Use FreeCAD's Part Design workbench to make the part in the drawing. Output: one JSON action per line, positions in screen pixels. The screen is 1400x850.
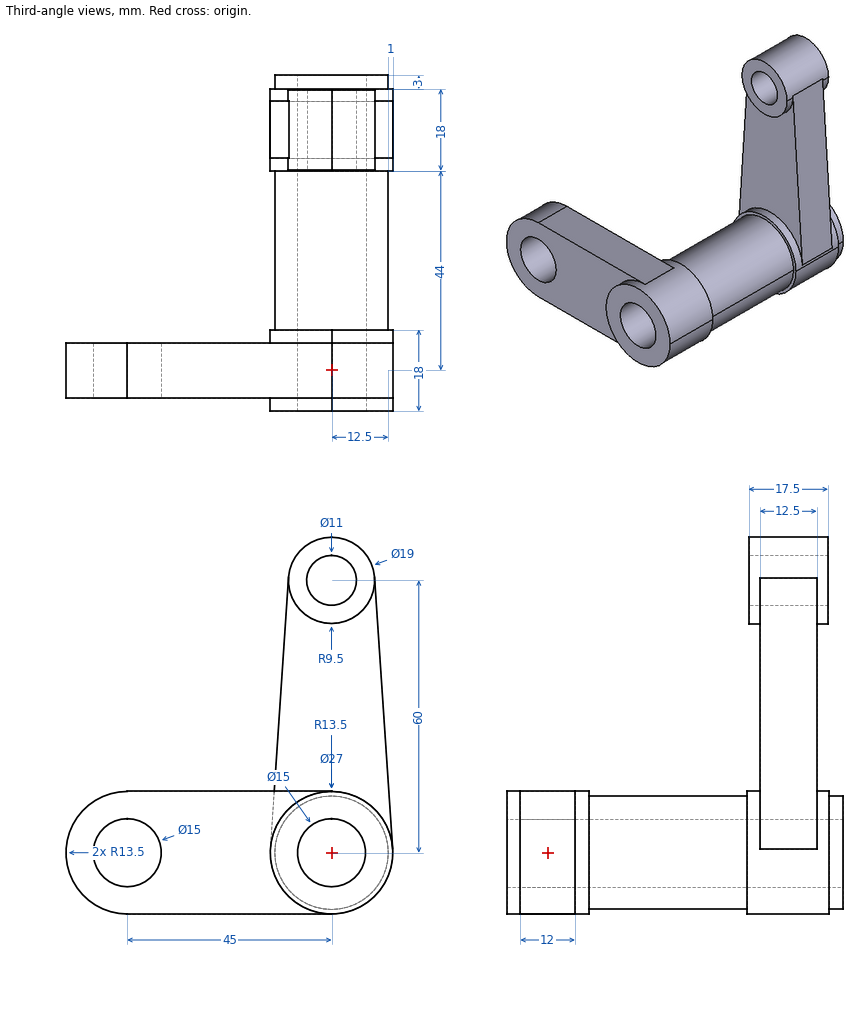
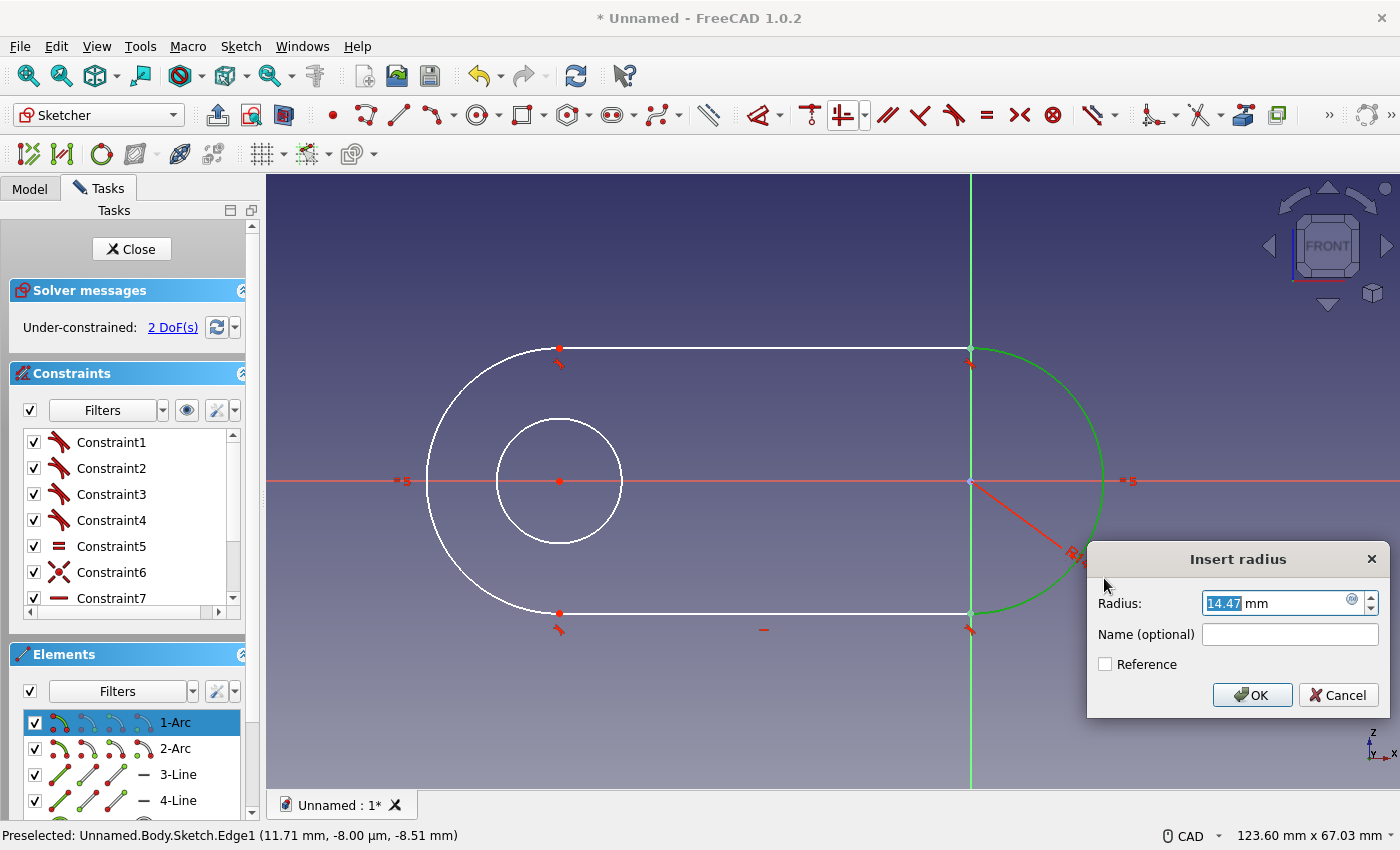
{"action": "type", "text": "13.5"}
{"action": "key", "text": "Return"}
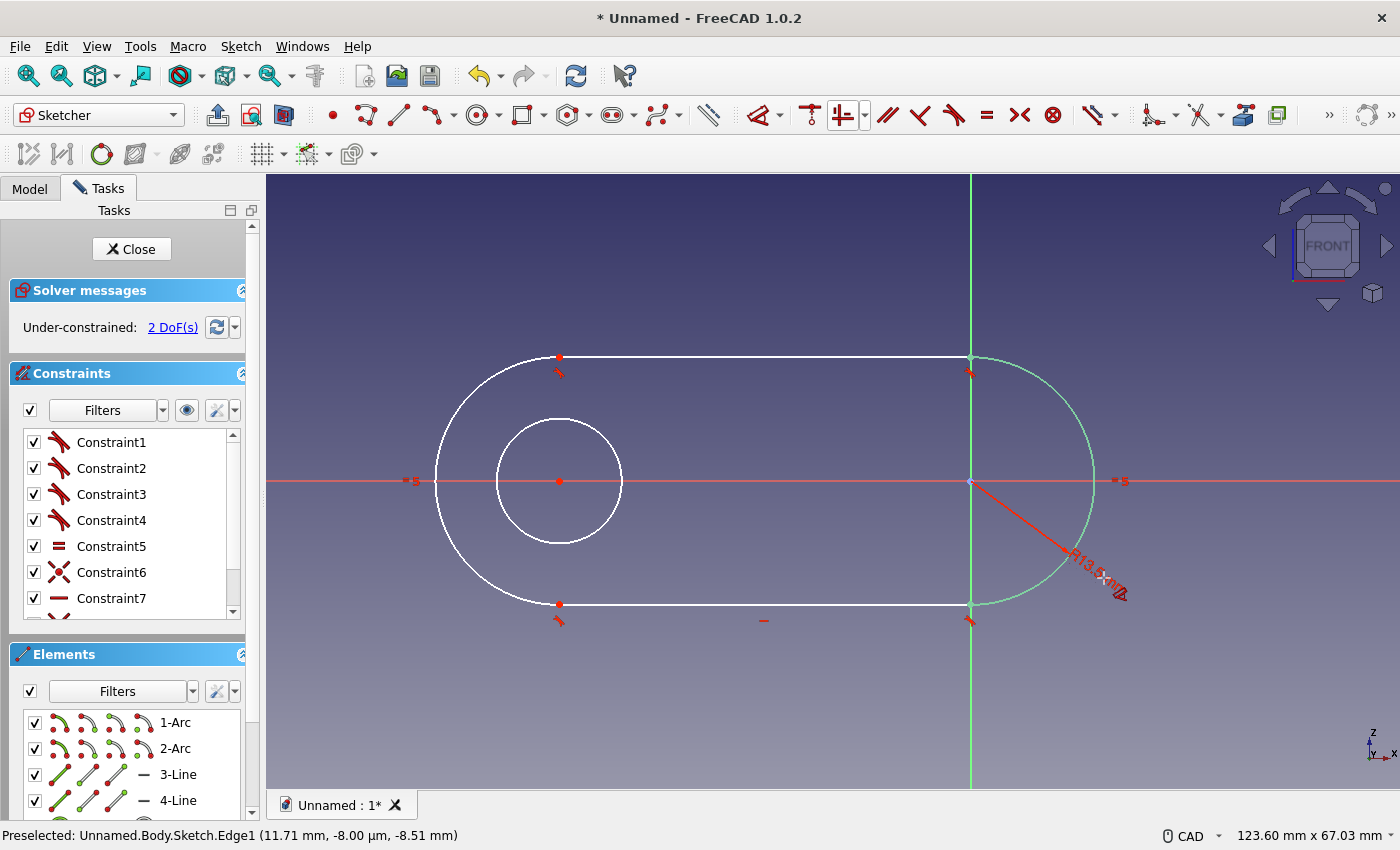
{"action": "left_click", "coordinate": [603, 437]}
{"action": "left_click", "coordinate": [626, 414]}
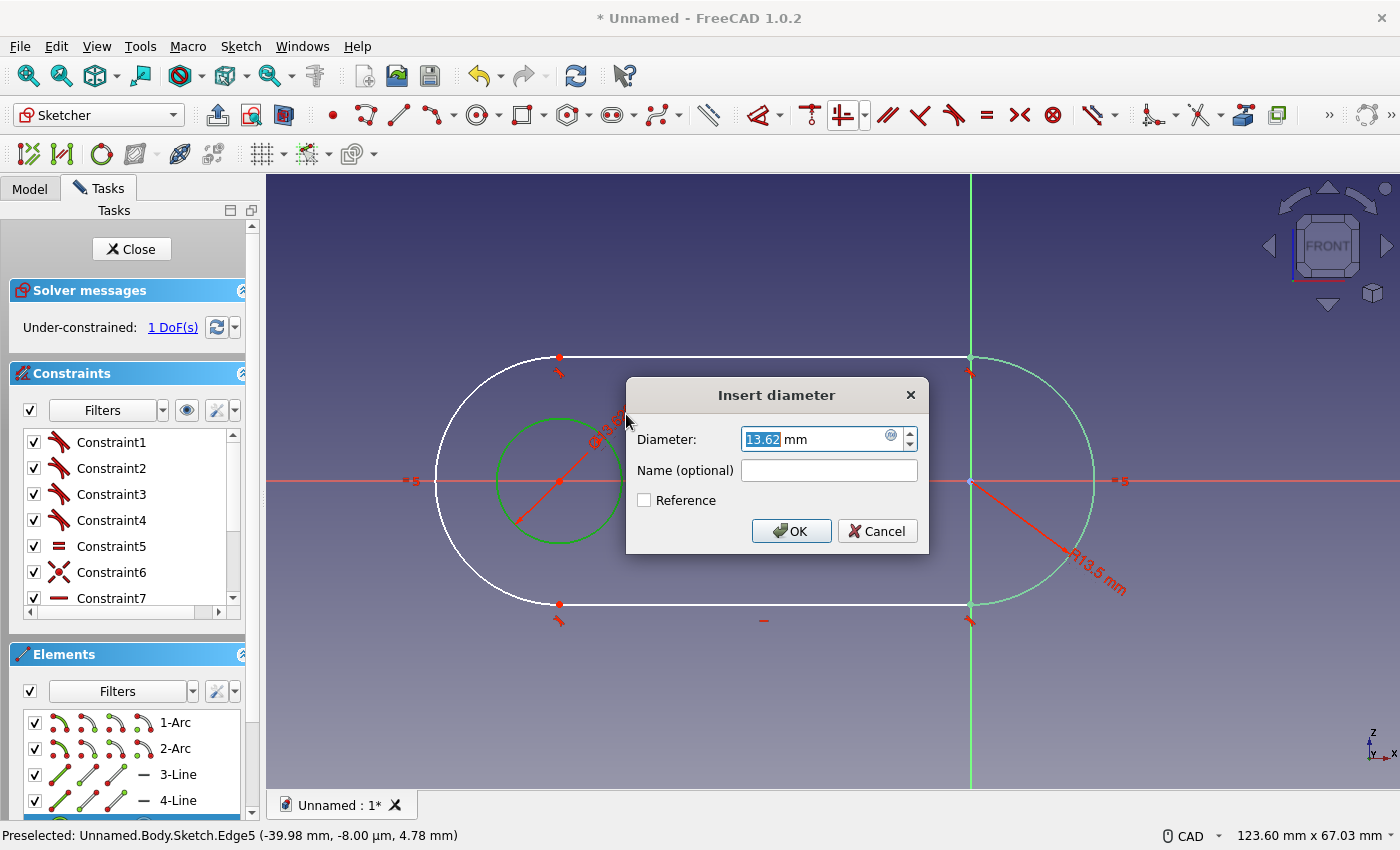
{"action": "type", "text": "15"}
{"action": "key", "text": "Return"}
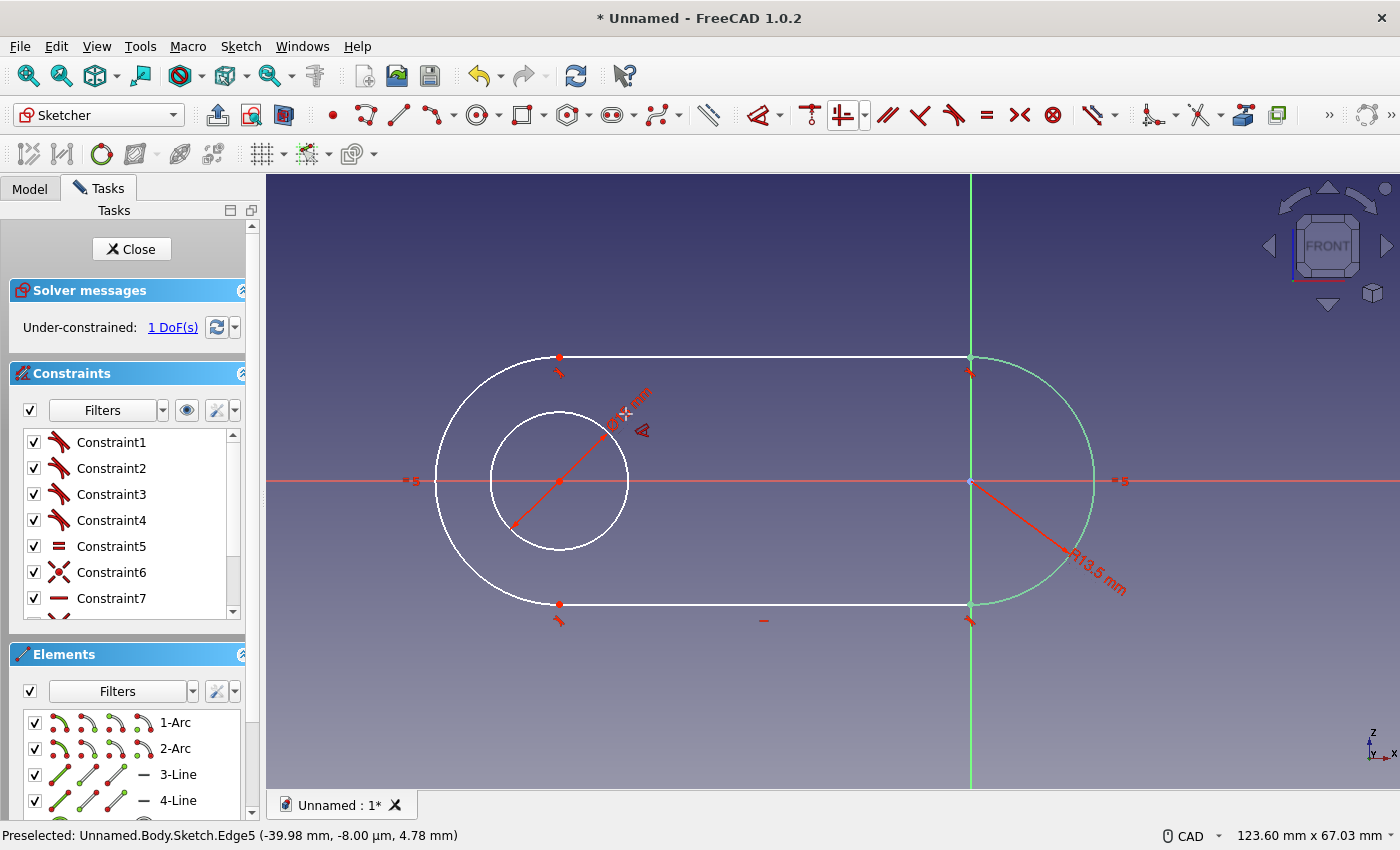
{"action": "left_click", "coordinate": [847, 605]}
{"action": "left_click", "coordinate": [765, 639]}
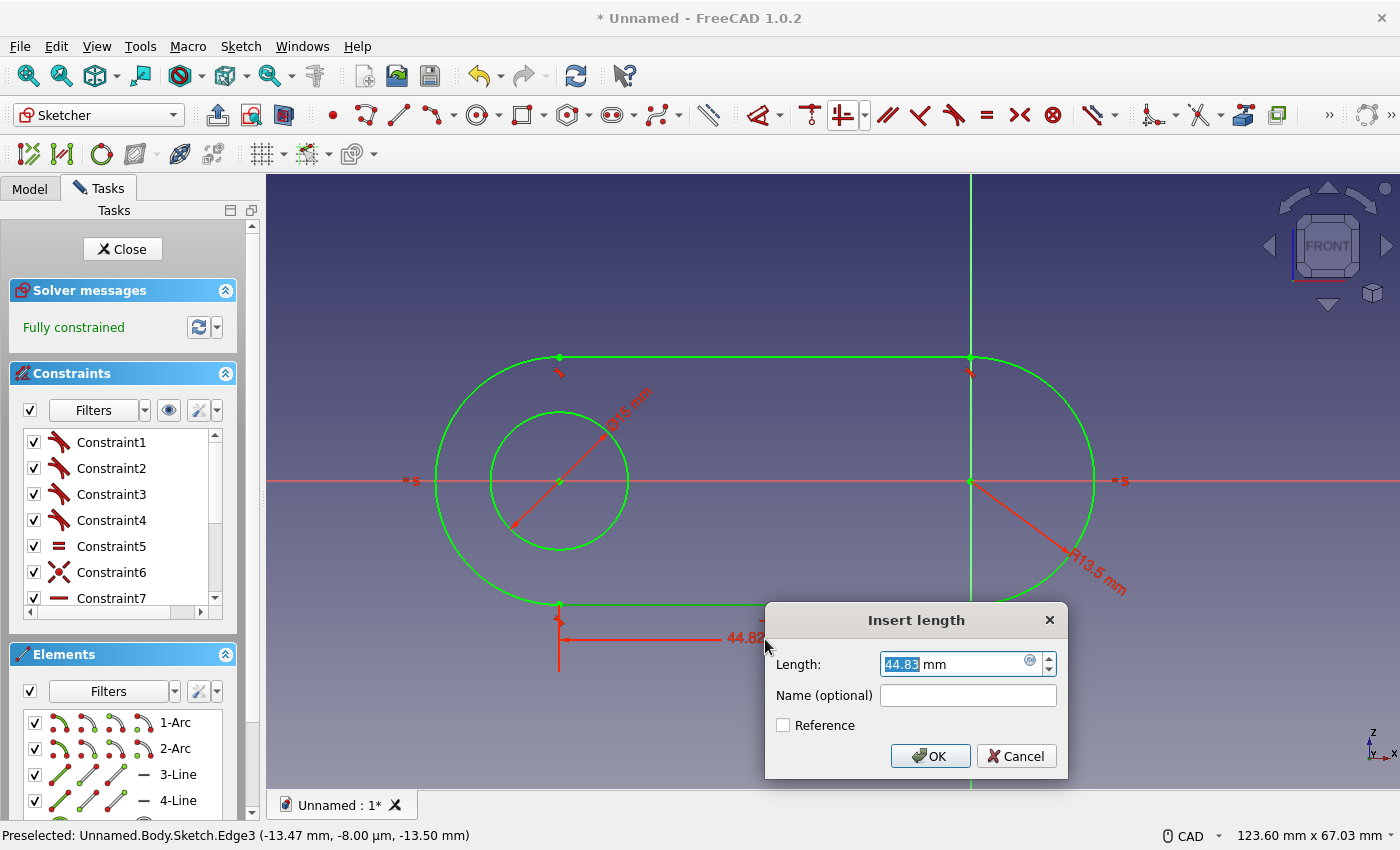
{"action": "type", "text": "45"}
{"action": "key", "text": "Return"}
{"action": "key", "text": "Escape"}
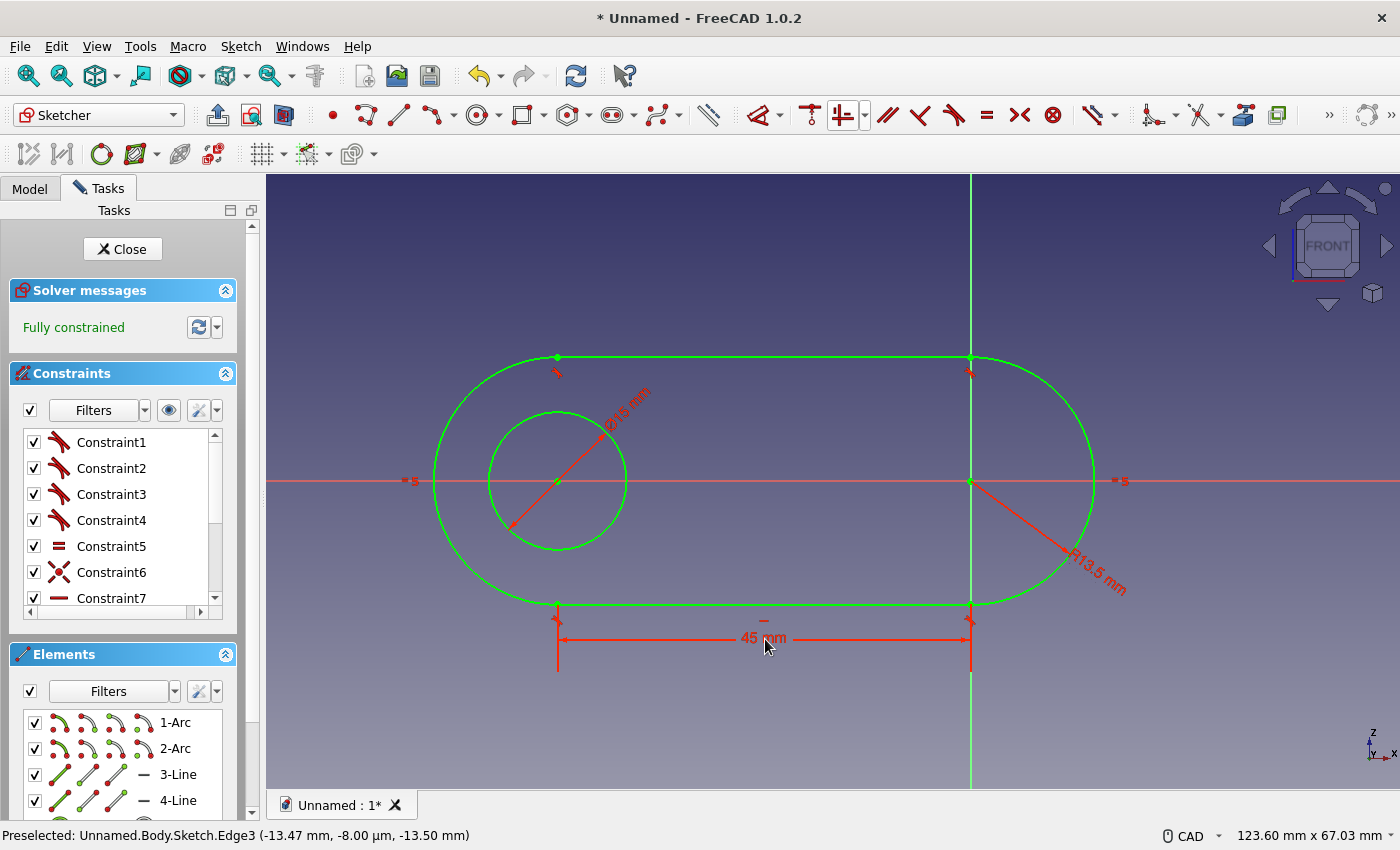
{"action": "left_click", "coordinate": [123, 249]}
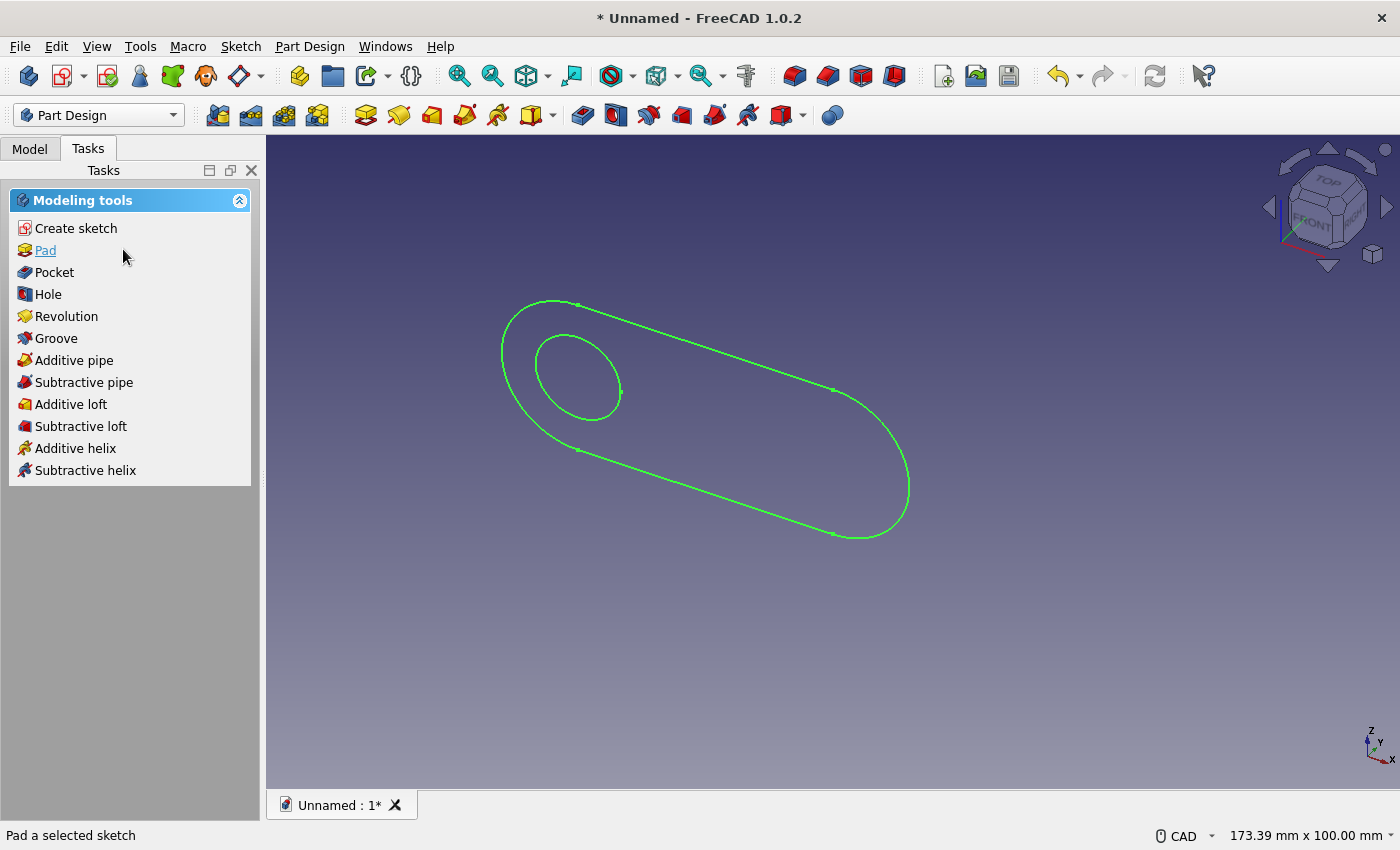
{"action": "left_click", "coordinate": [366, 116]}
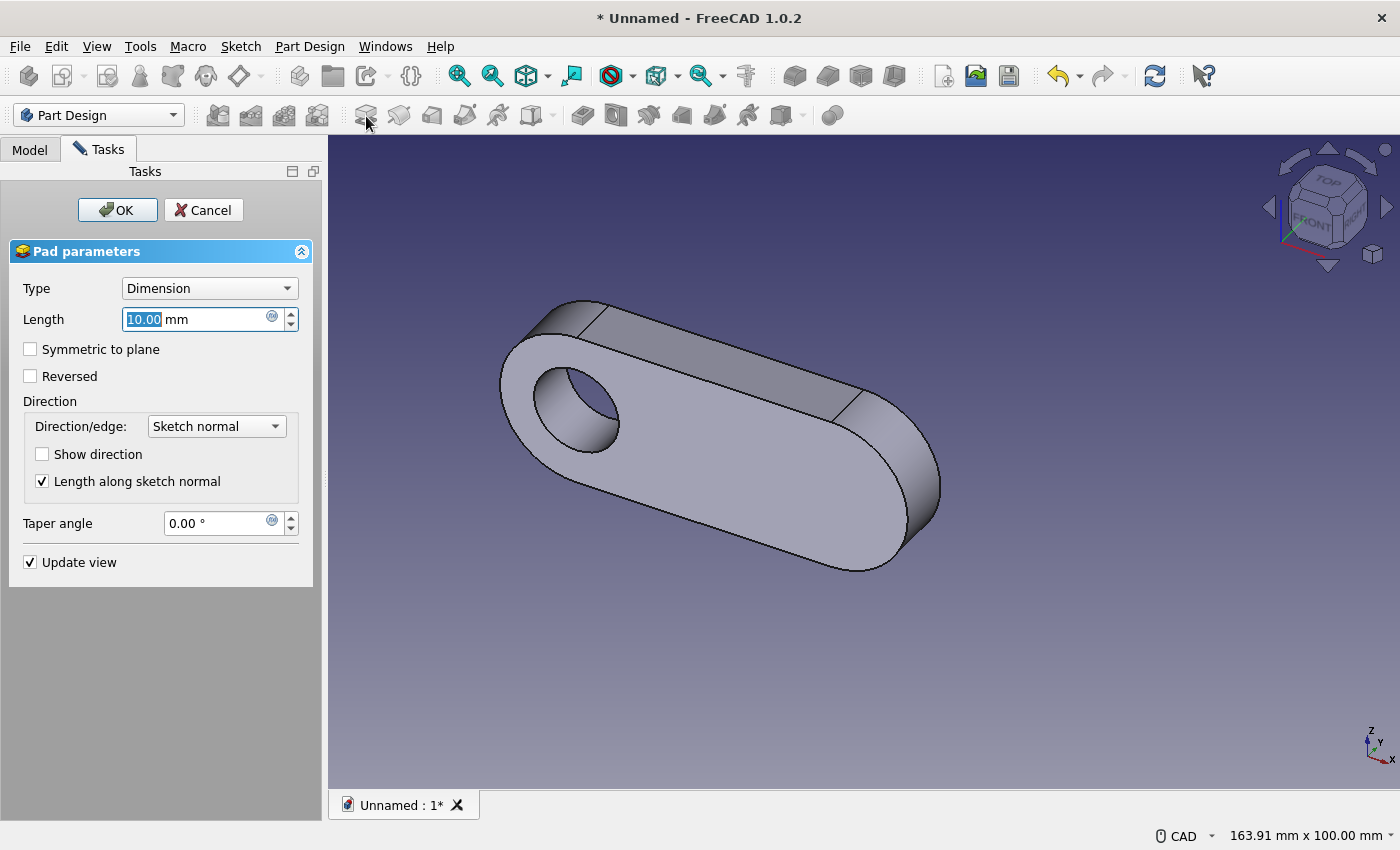
{"action": "type", "text": "12"}
{"action": "key", "text": "Tab"}